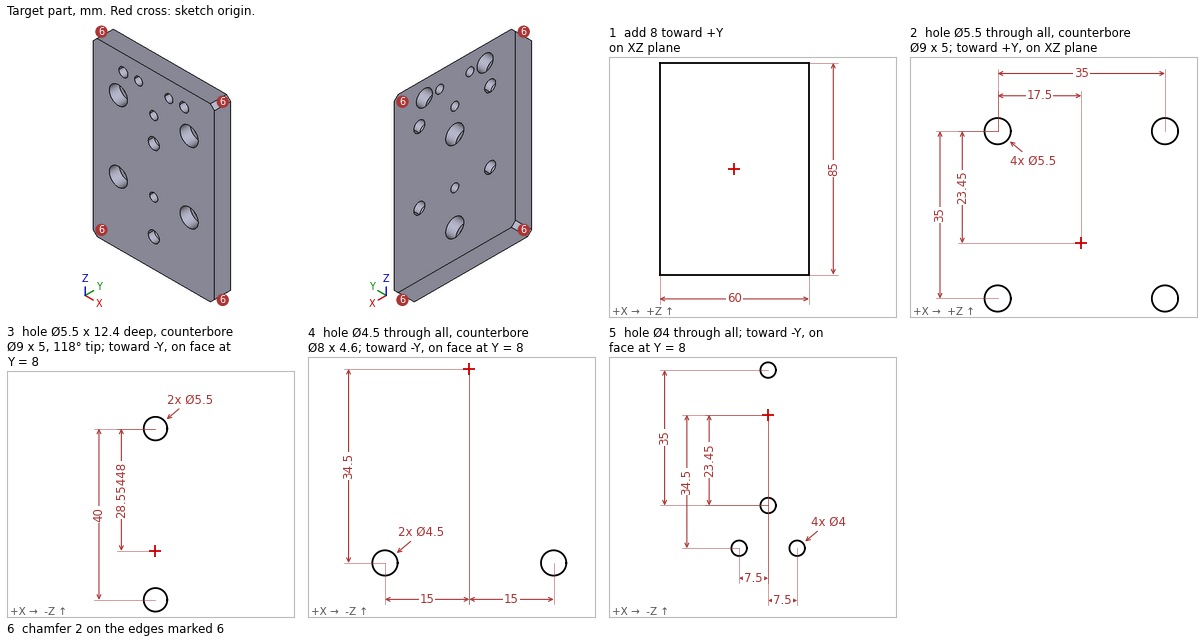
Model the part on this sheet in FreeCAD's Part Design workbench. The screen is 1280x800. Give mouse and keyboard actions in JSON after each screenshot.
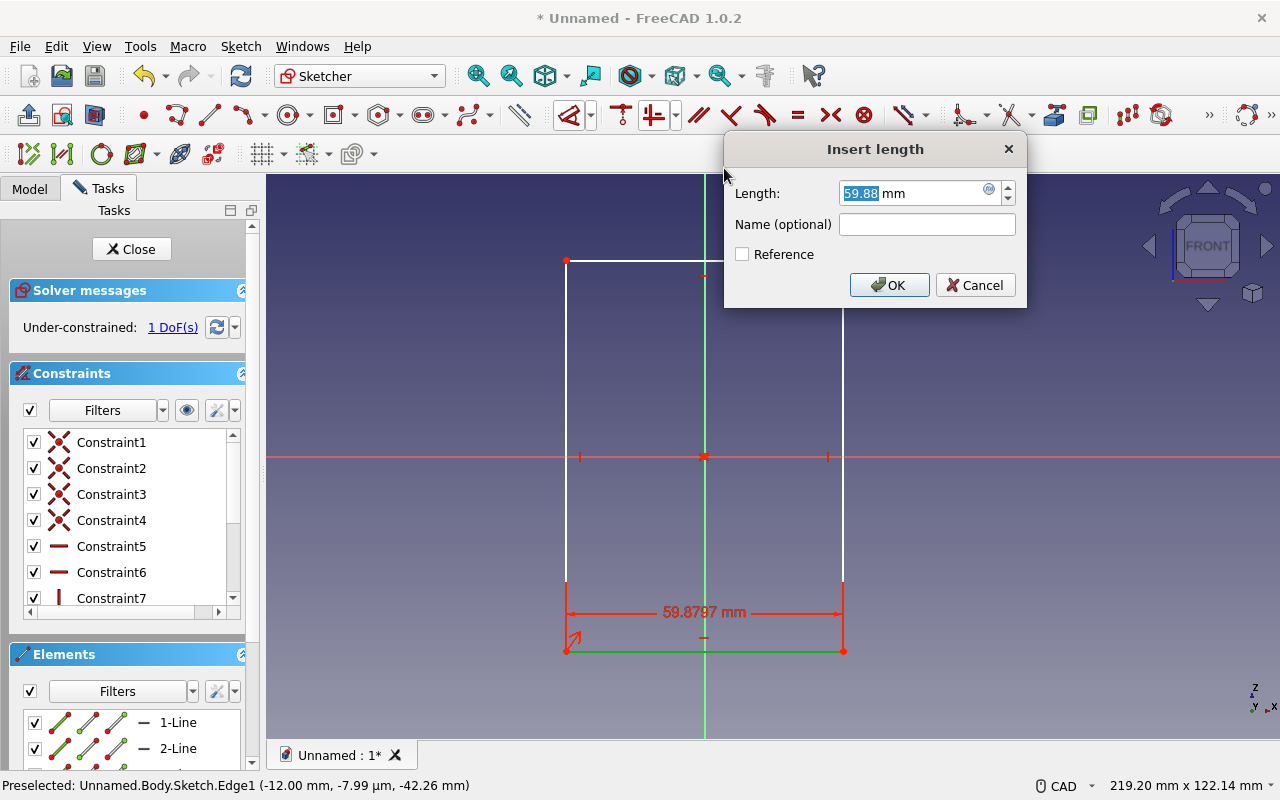
{"action": "type", "text": "60"}
{"action": "key", "text": "Return"}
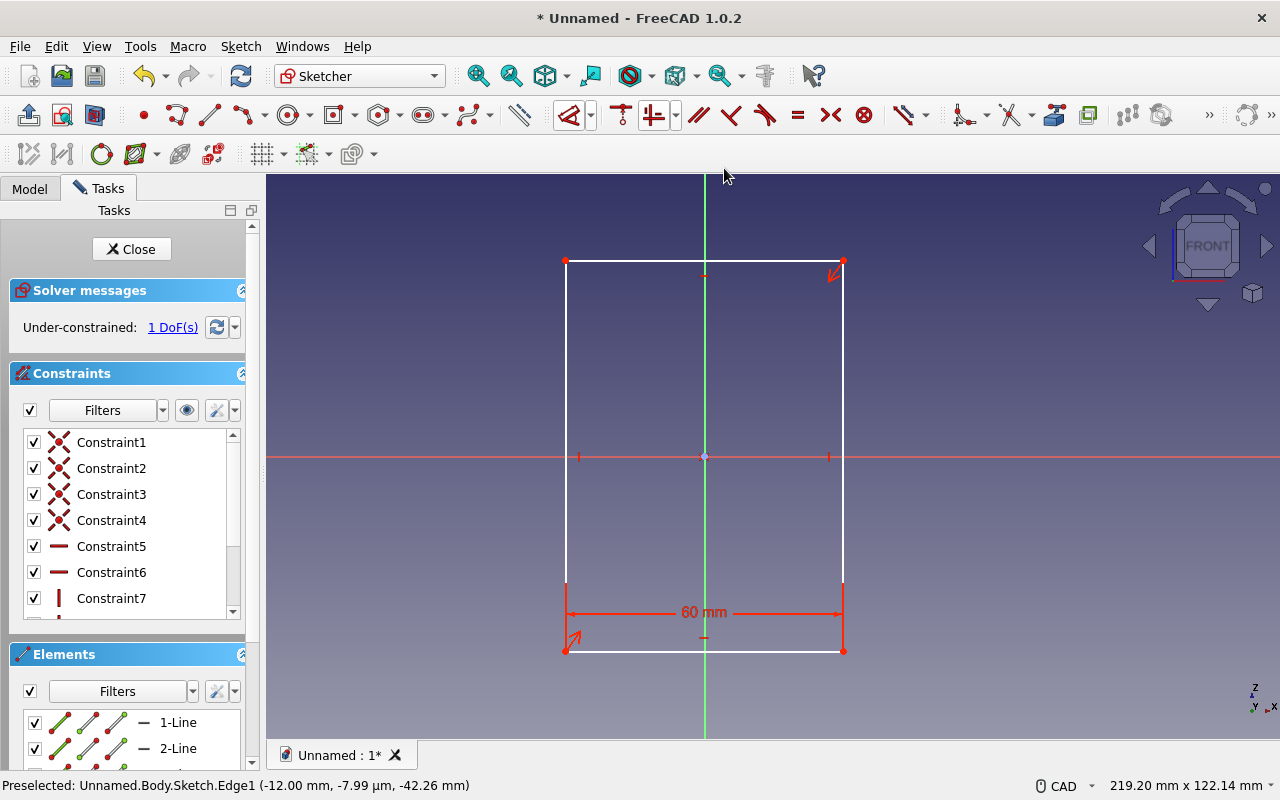
{"action": "left_click", "coordinate": [843, 535]}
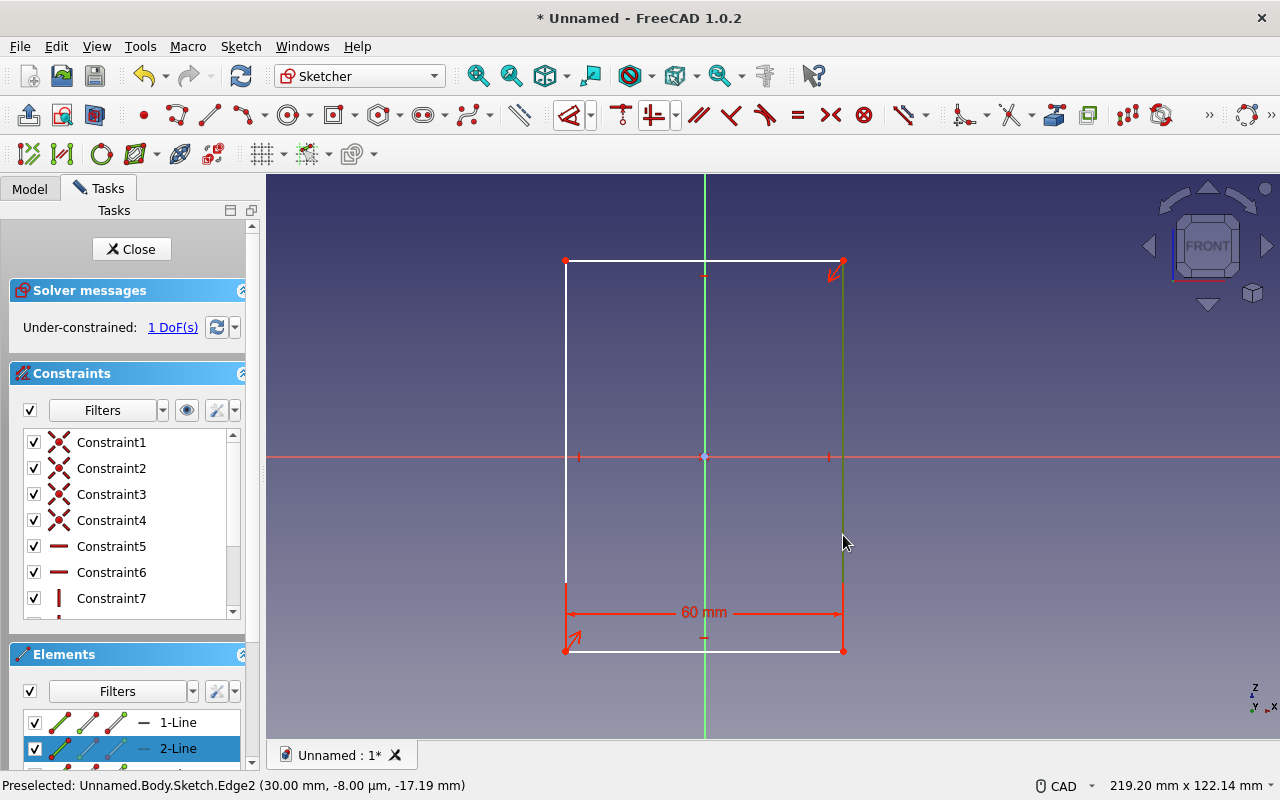
{"action": "key", "text": "i"}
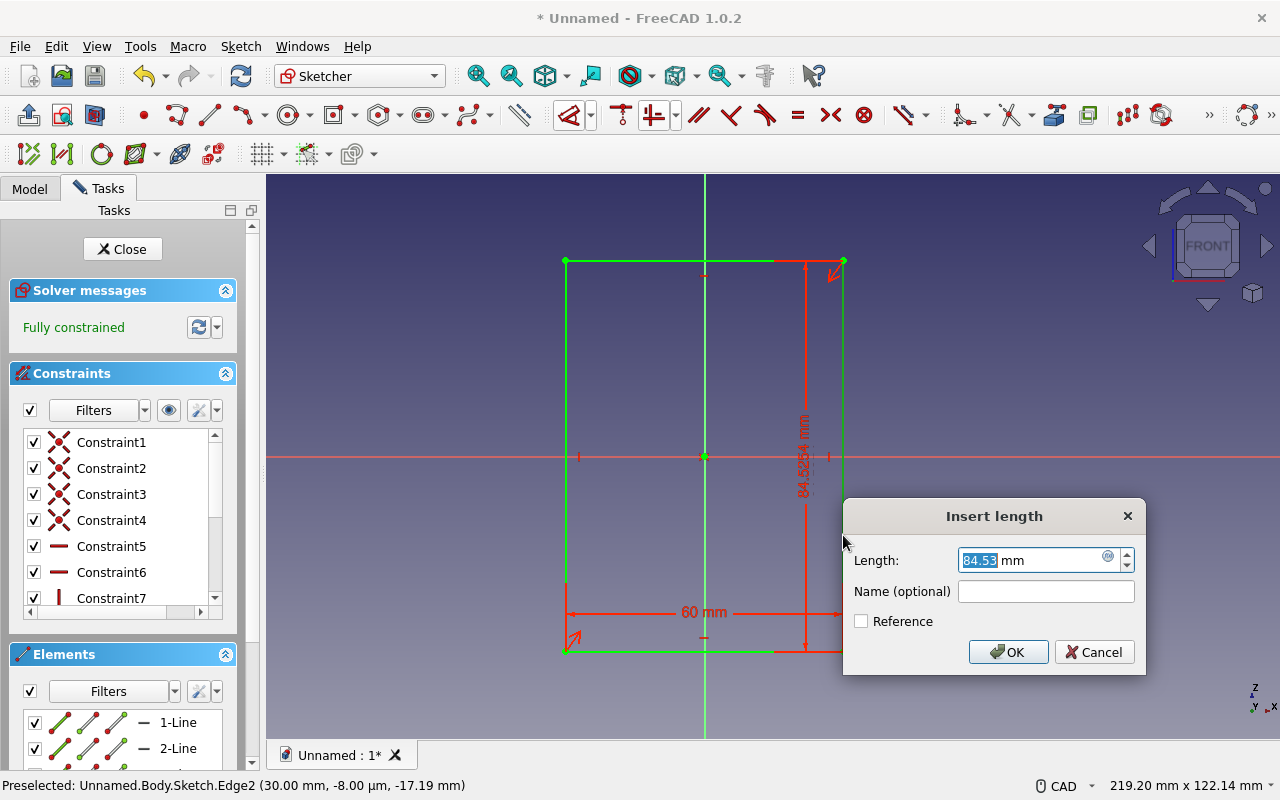
{"action": "type", "text": "85"}
{"action": "key", "text": "Return"}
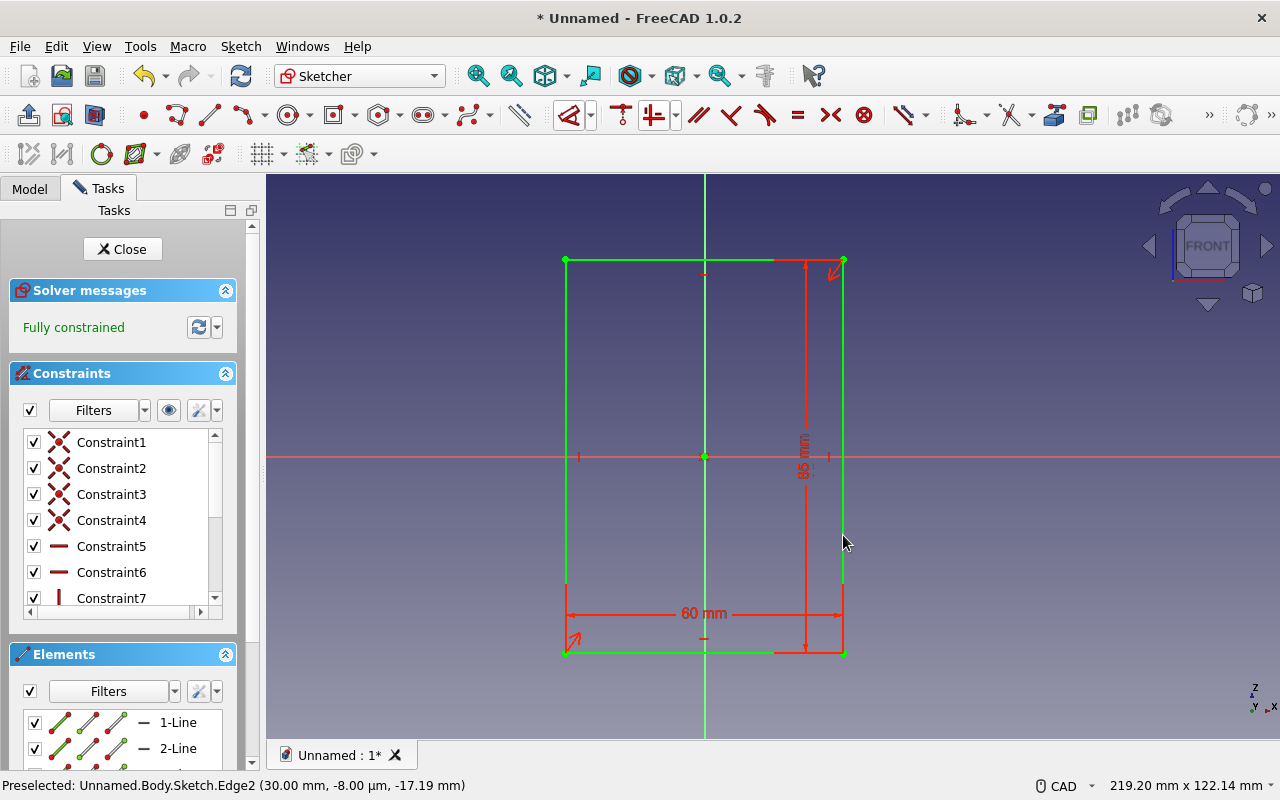
{"action": "left_click", "coordinate": [123, 249]}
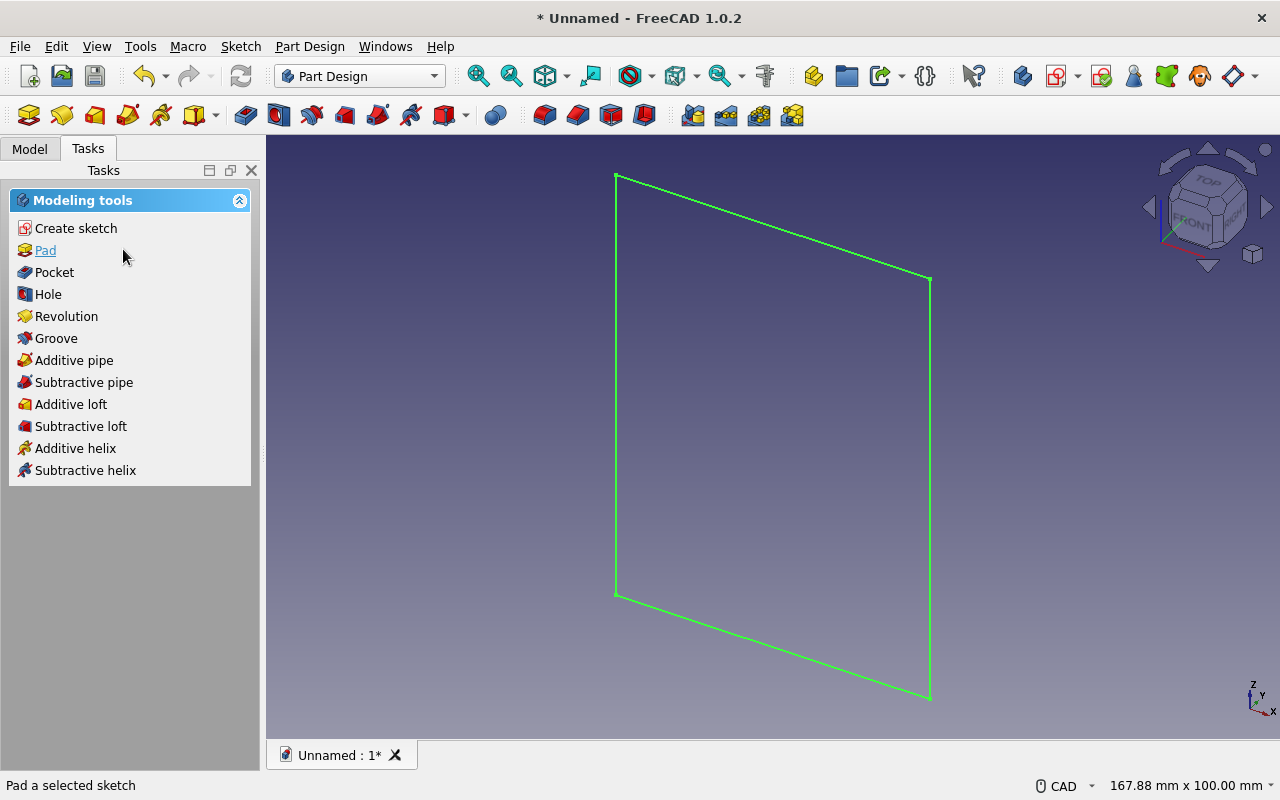
{"action": "left_click", "coordinate": [29, 116]}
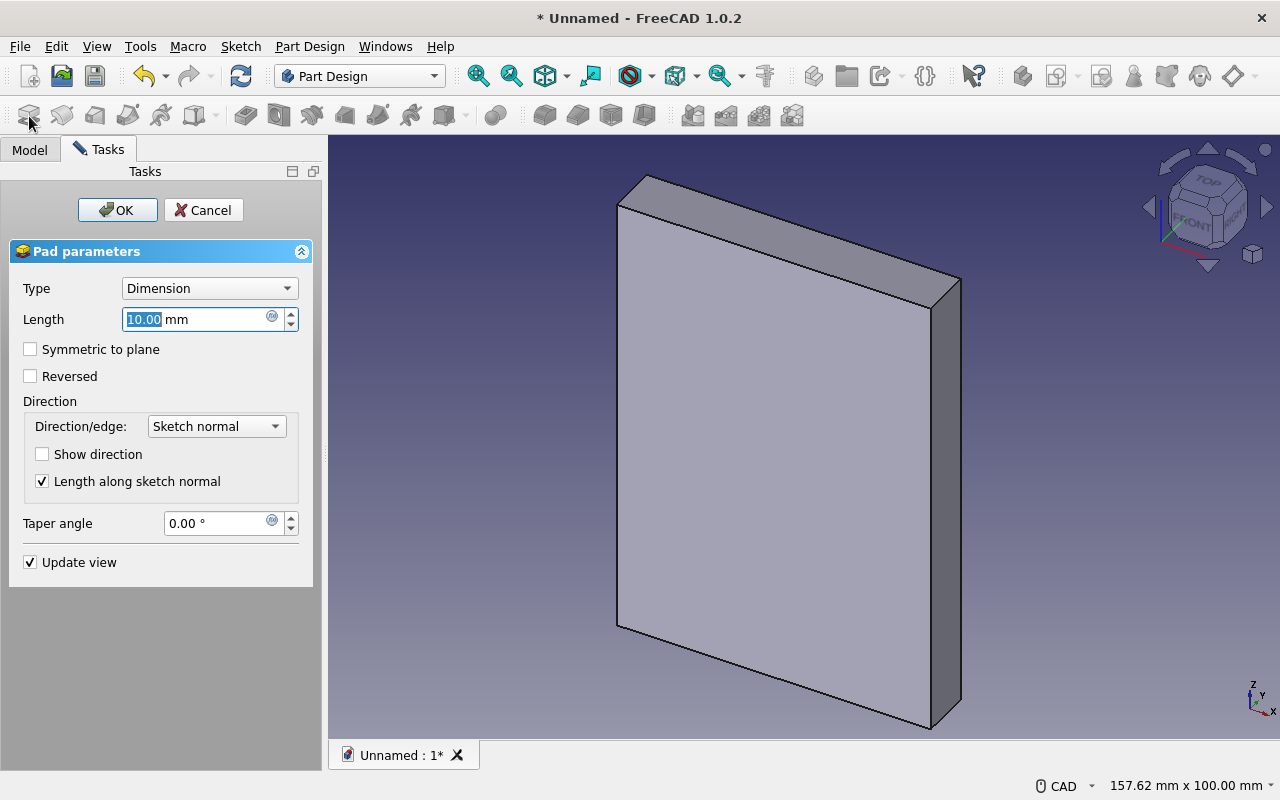
{"action": "type", "text": "8"}
{"action": "key", "text": "Tab"}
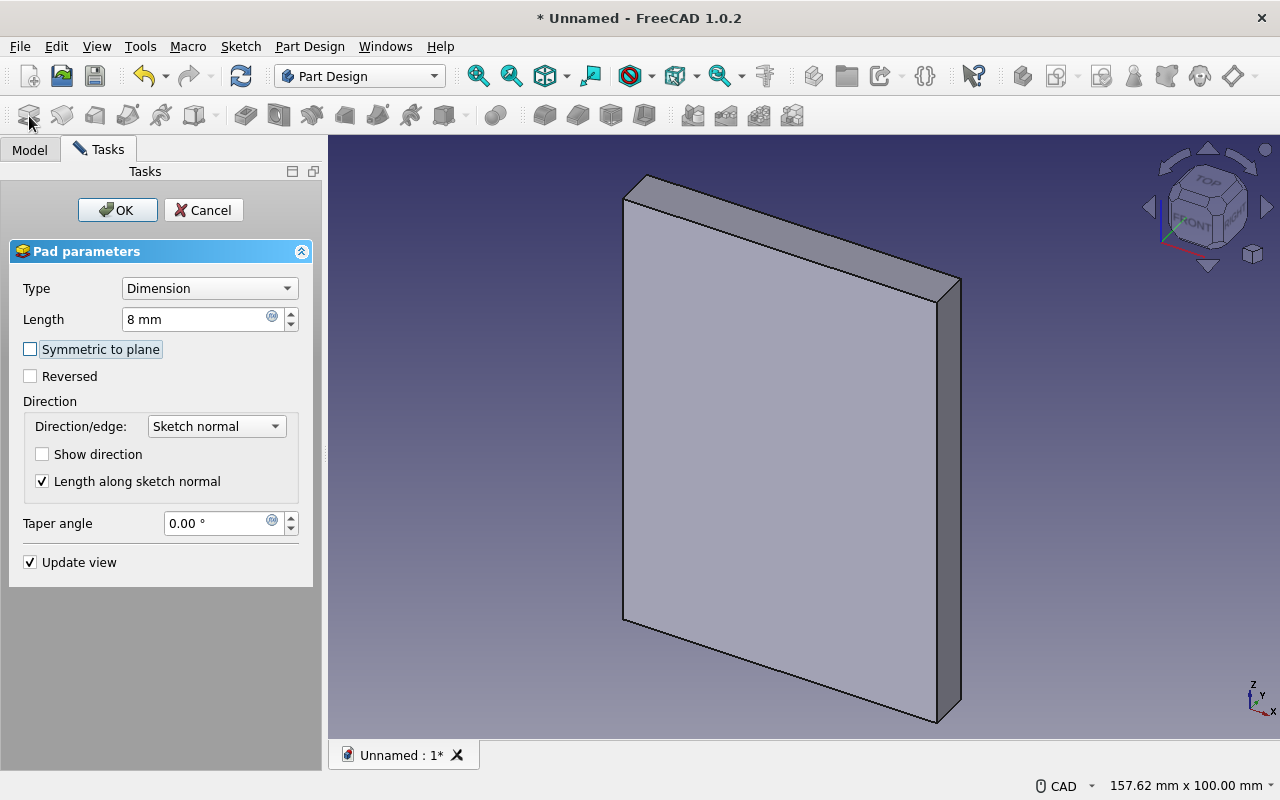
{"action": "left_click", "coordinate": [31, 376]}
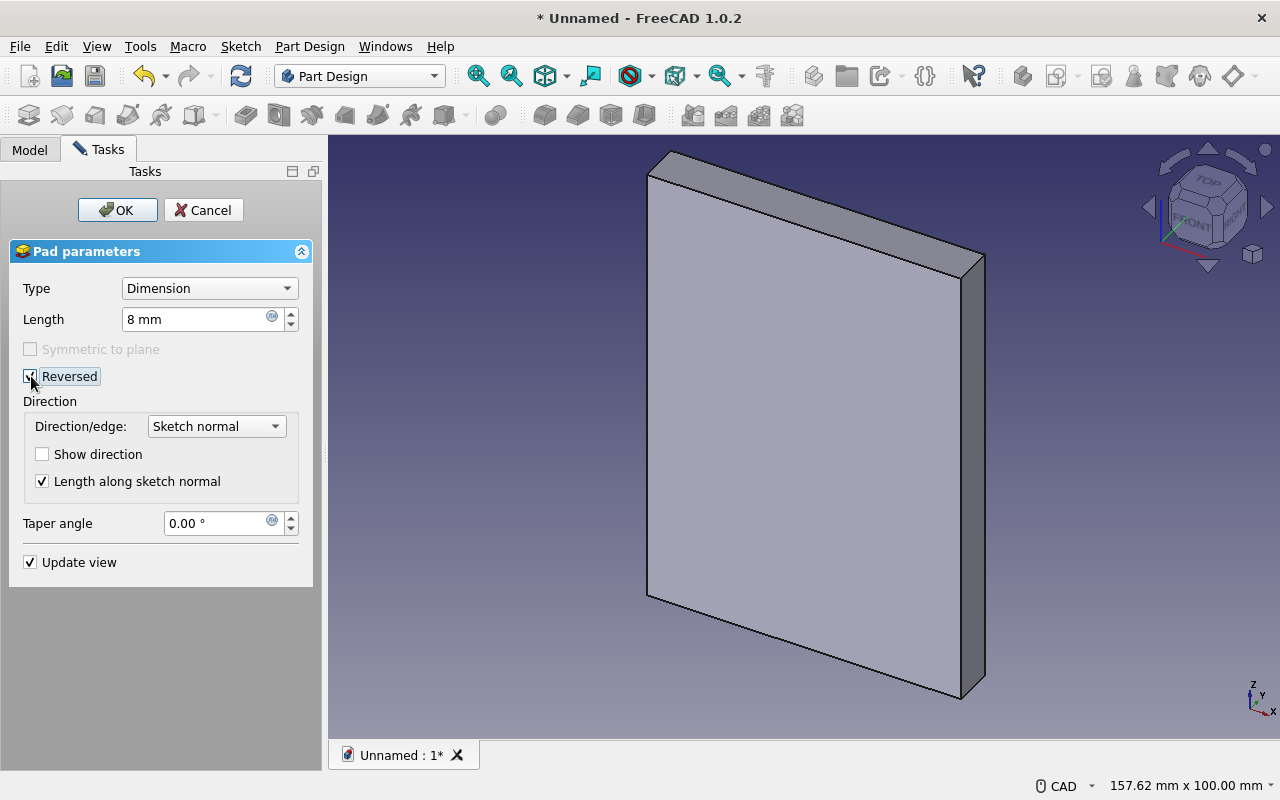
{"action": "left_click", "coordinate": [118, 210]}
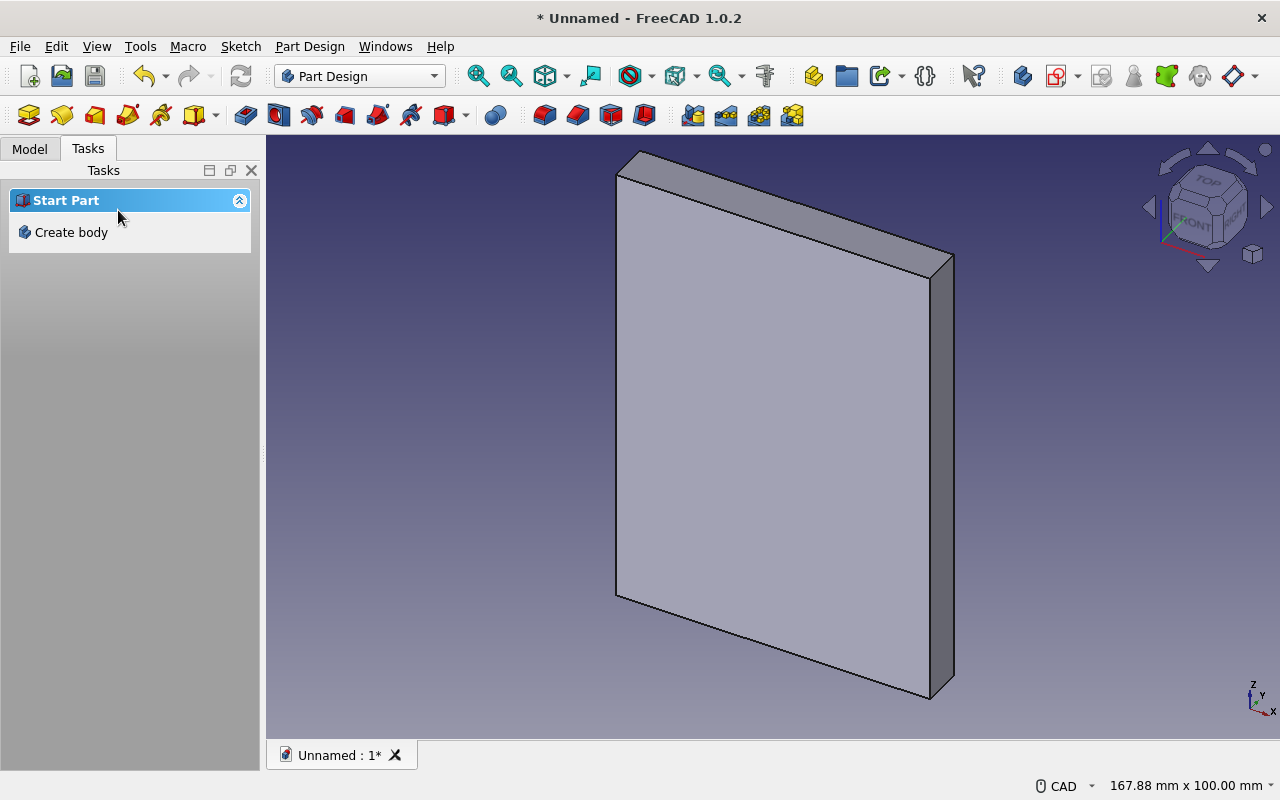
{"action": "left_click", "coordinate": [1056, 76]}